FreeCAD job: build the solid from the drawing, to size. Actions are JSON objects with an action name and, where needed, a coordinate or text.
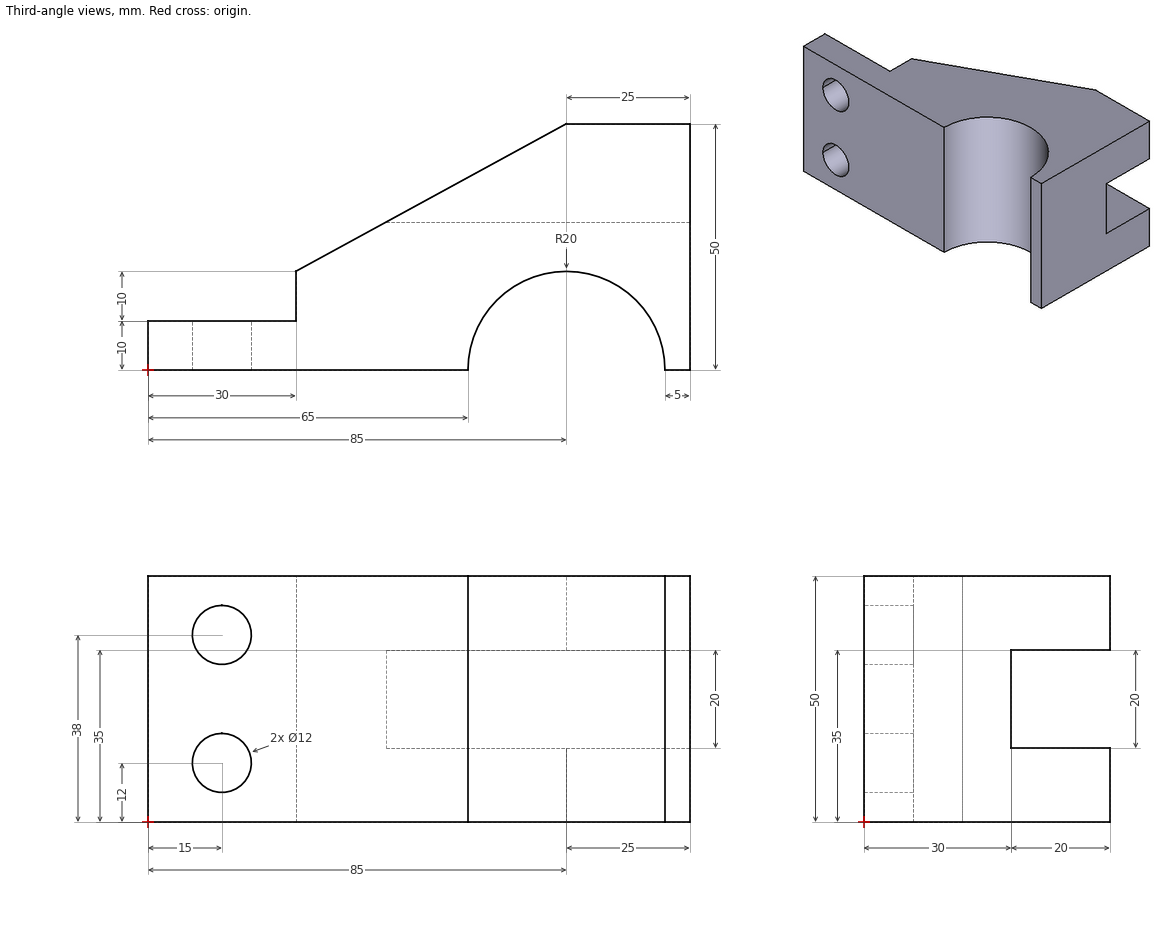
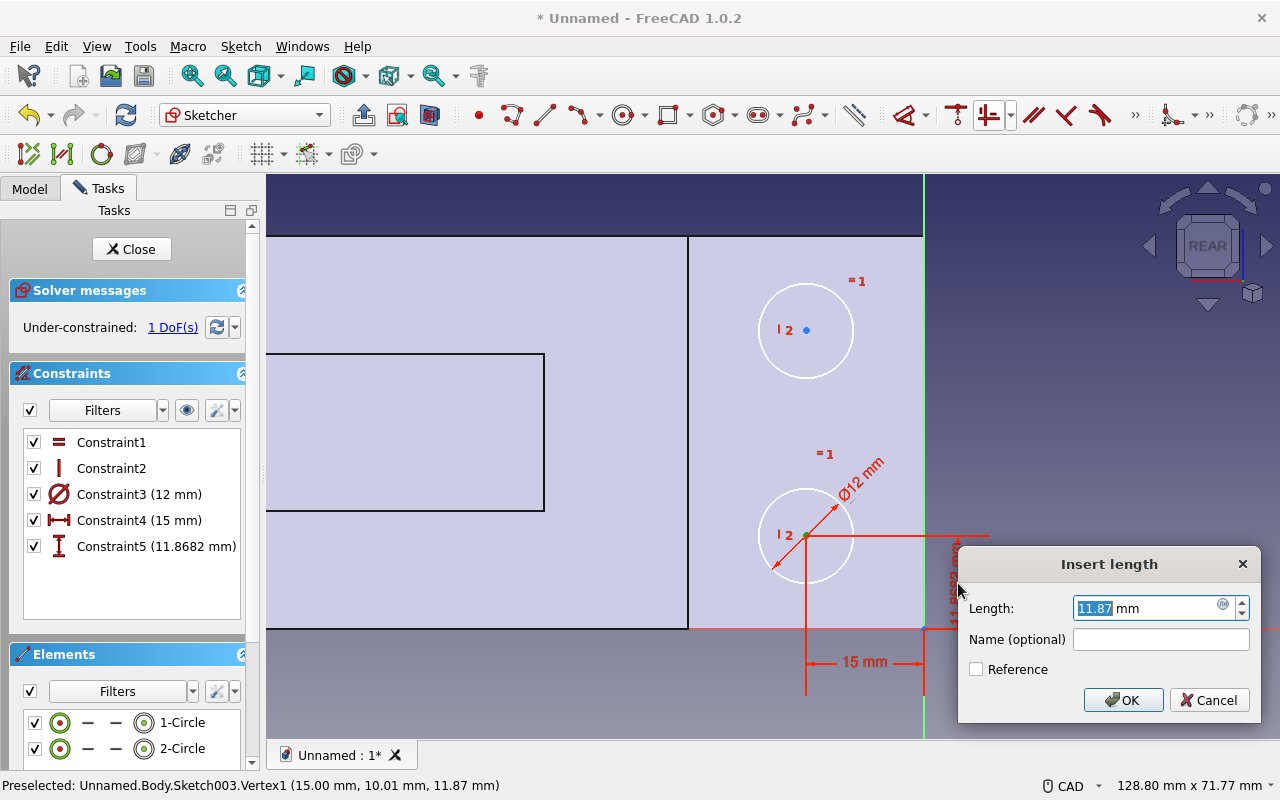
{"action": "type", "text": "12"}
{"action": "key", "text": "Return"}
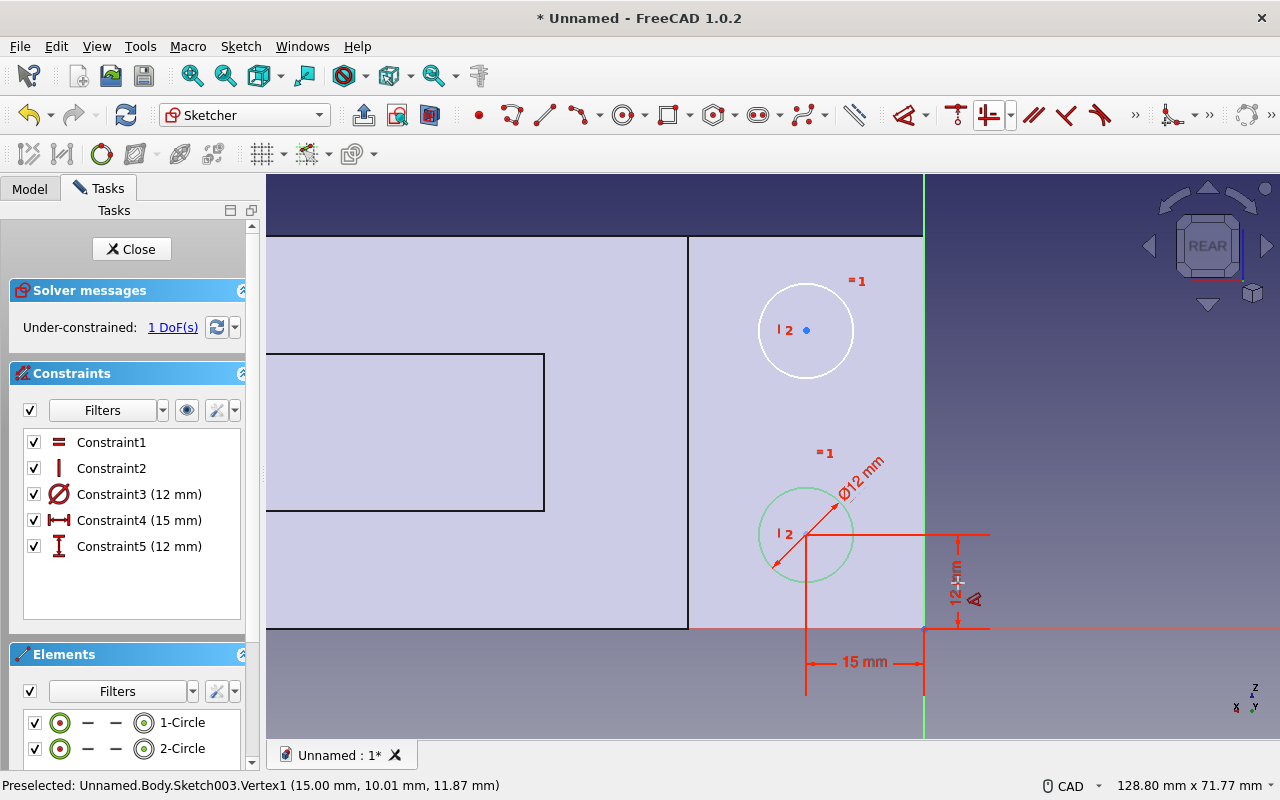
{"action": "left_click", "coordinate": [806, 331]}
{"action": "left_click", "coordinate": [958, 480]}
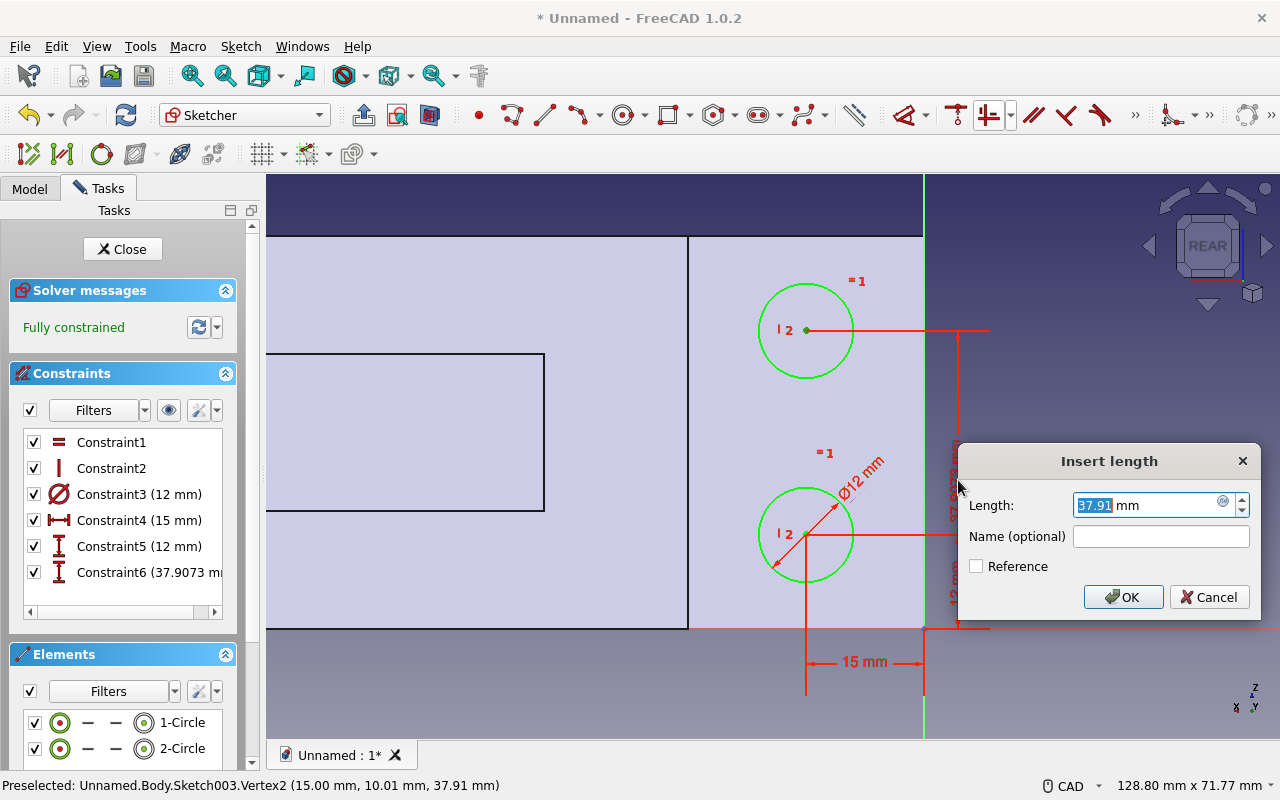
{"action": "type", "text": "38"}
{"action": "key", "text": "Return"}
{"action": "key", "text": "Escape"}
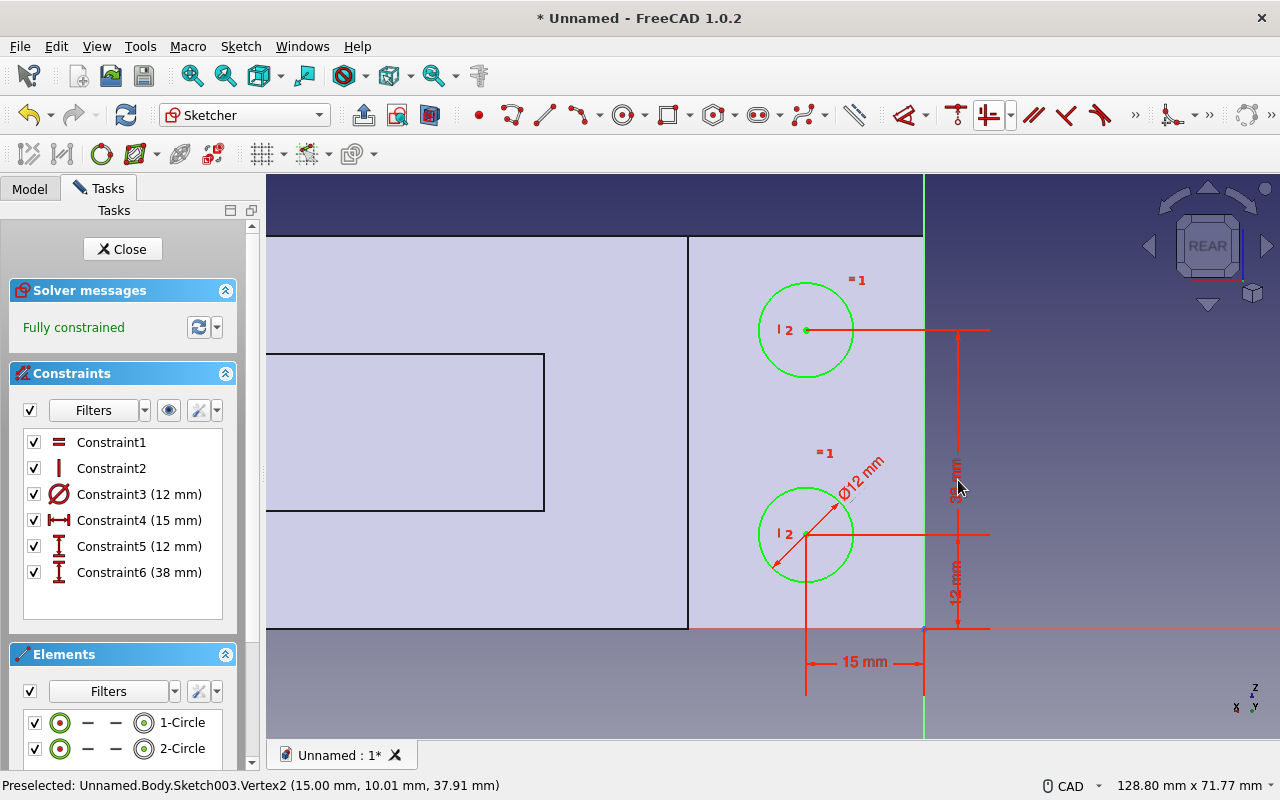
{"action": "left_click", "coordinate": [123, 249]}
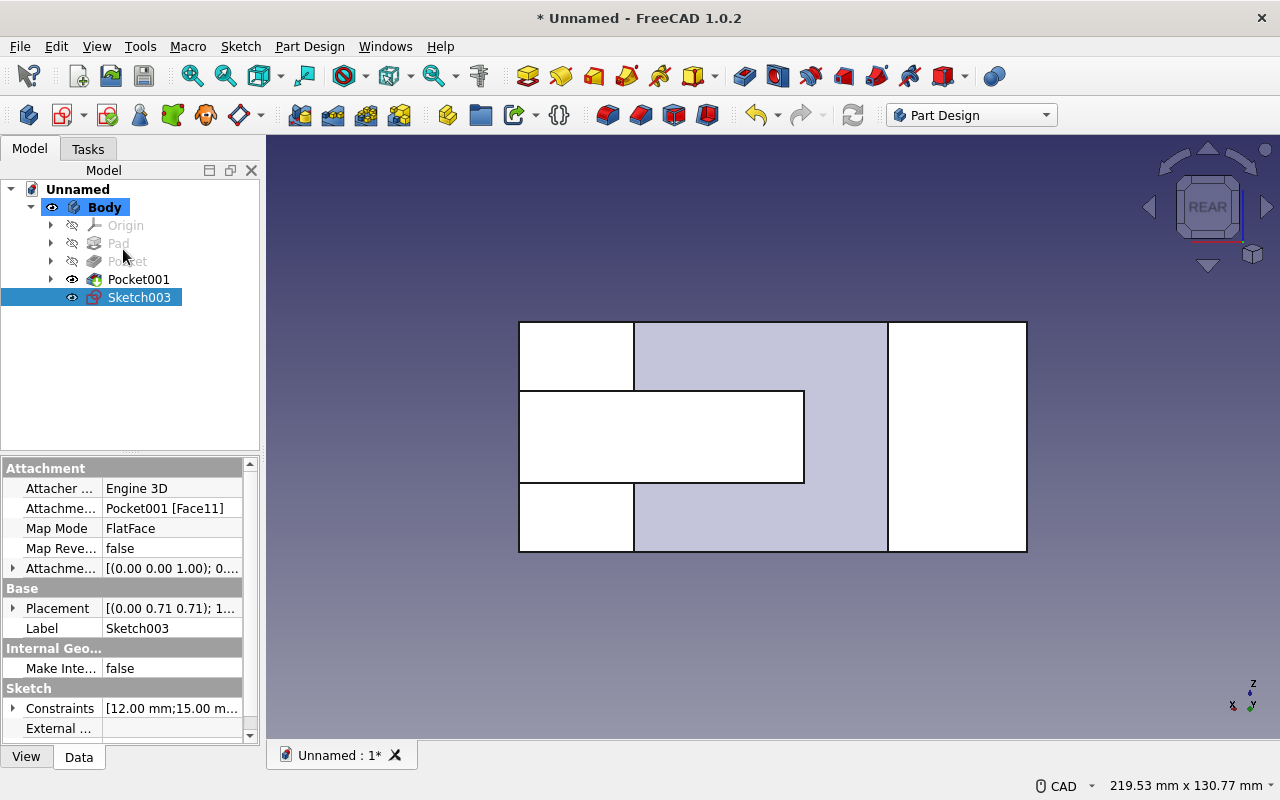
{"action": "left_click", "coordinate": [745, 76]}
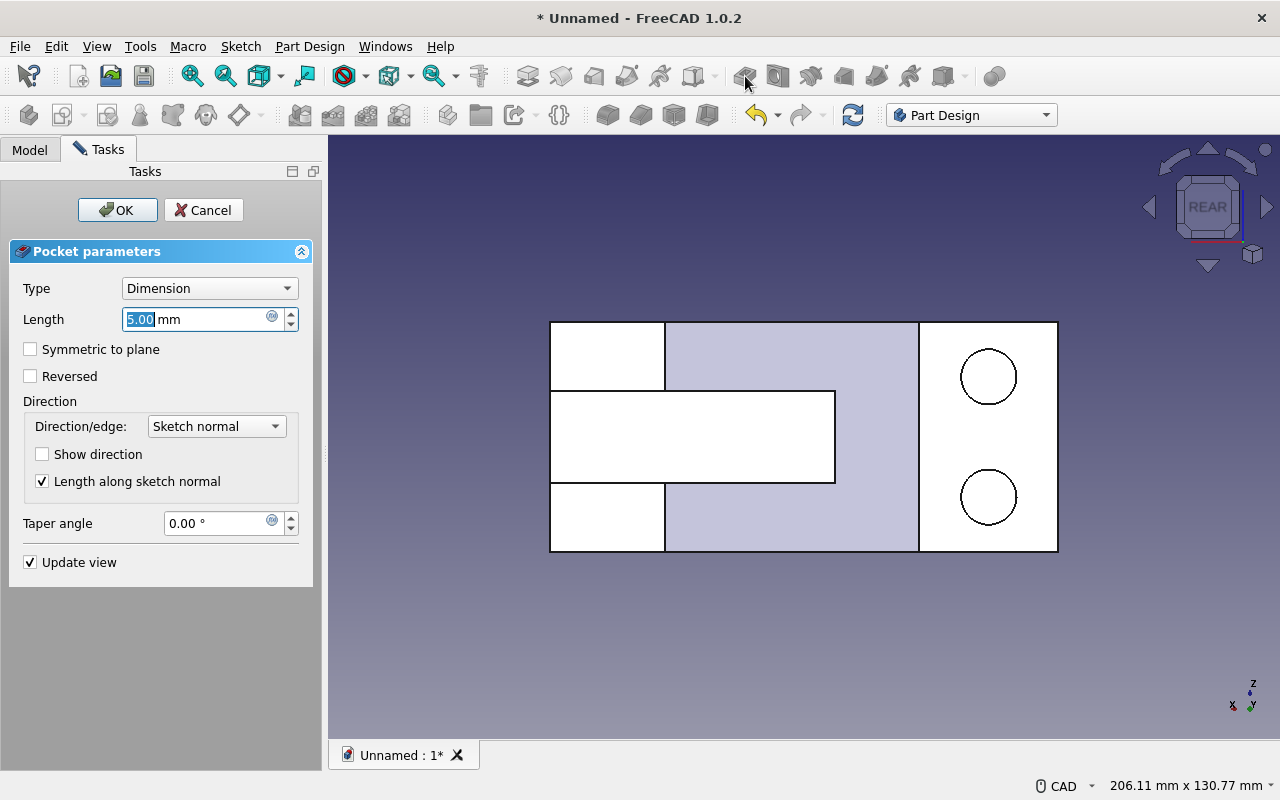
{"action": "left_click", "coordinate": [210, 288]}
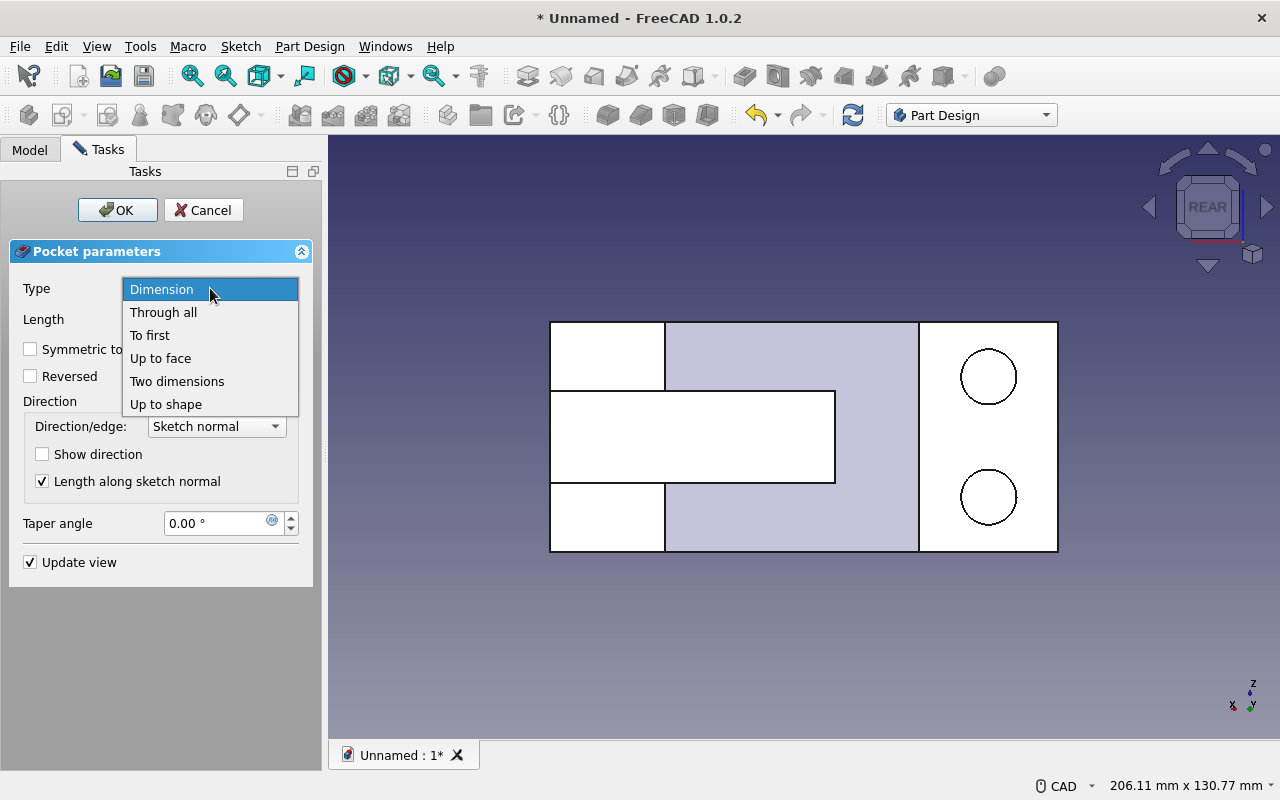
{"action": "left_click", "coordinate": [208, 312]}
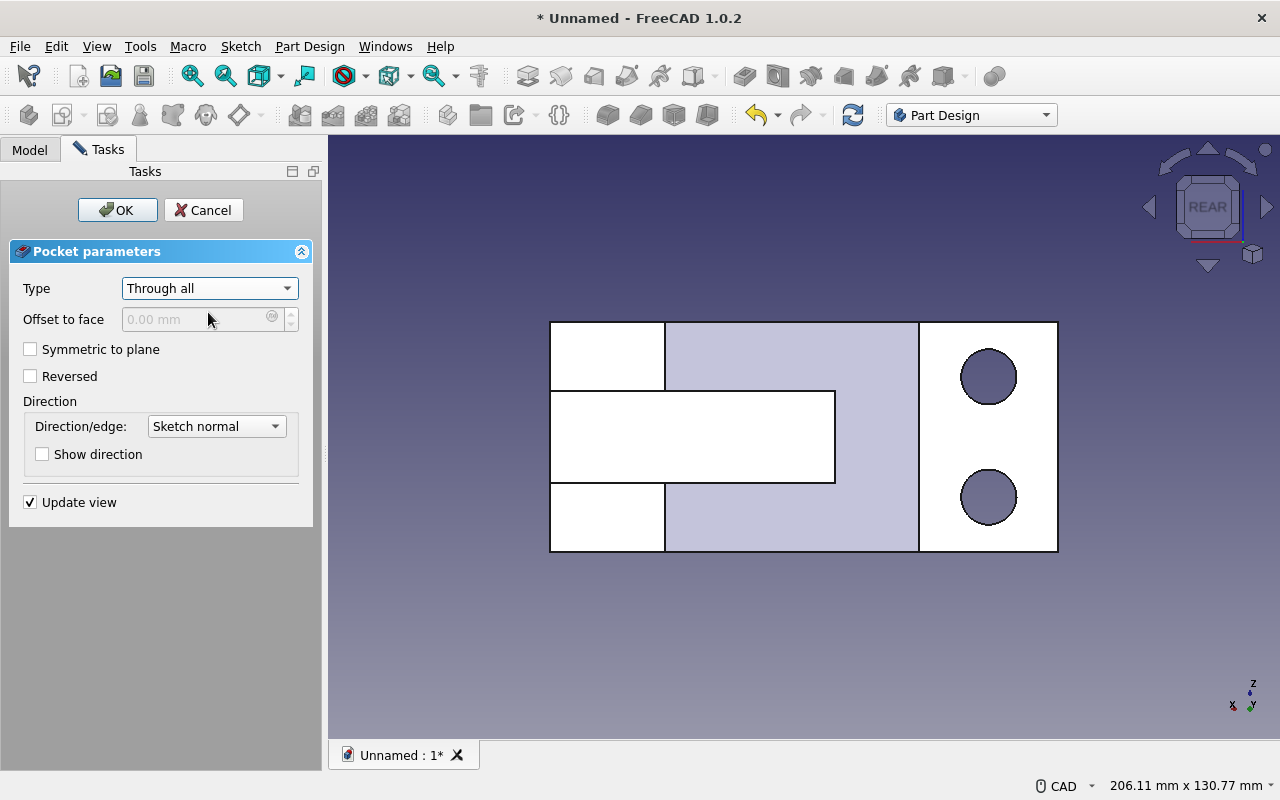
{"action": "left_click", "coordinate": [118, 210]}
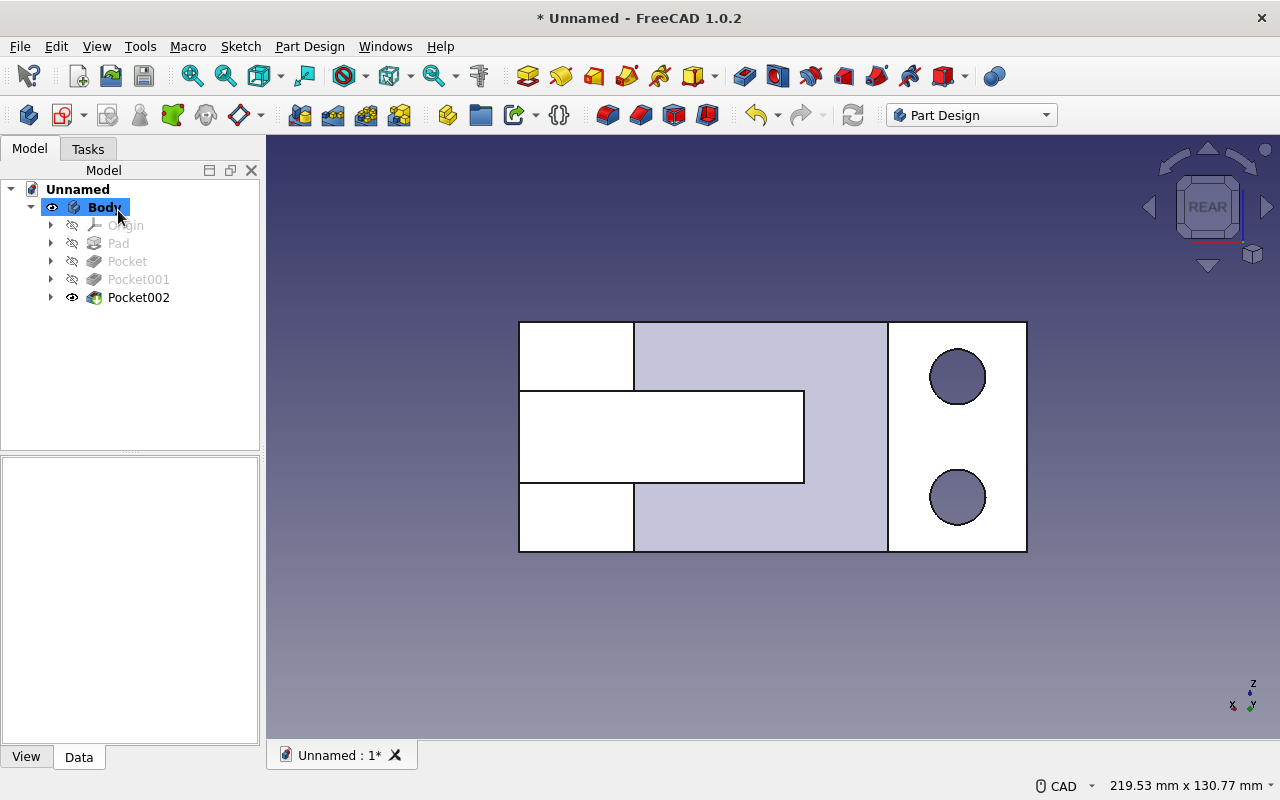
{"action": "key", "text": "0"}